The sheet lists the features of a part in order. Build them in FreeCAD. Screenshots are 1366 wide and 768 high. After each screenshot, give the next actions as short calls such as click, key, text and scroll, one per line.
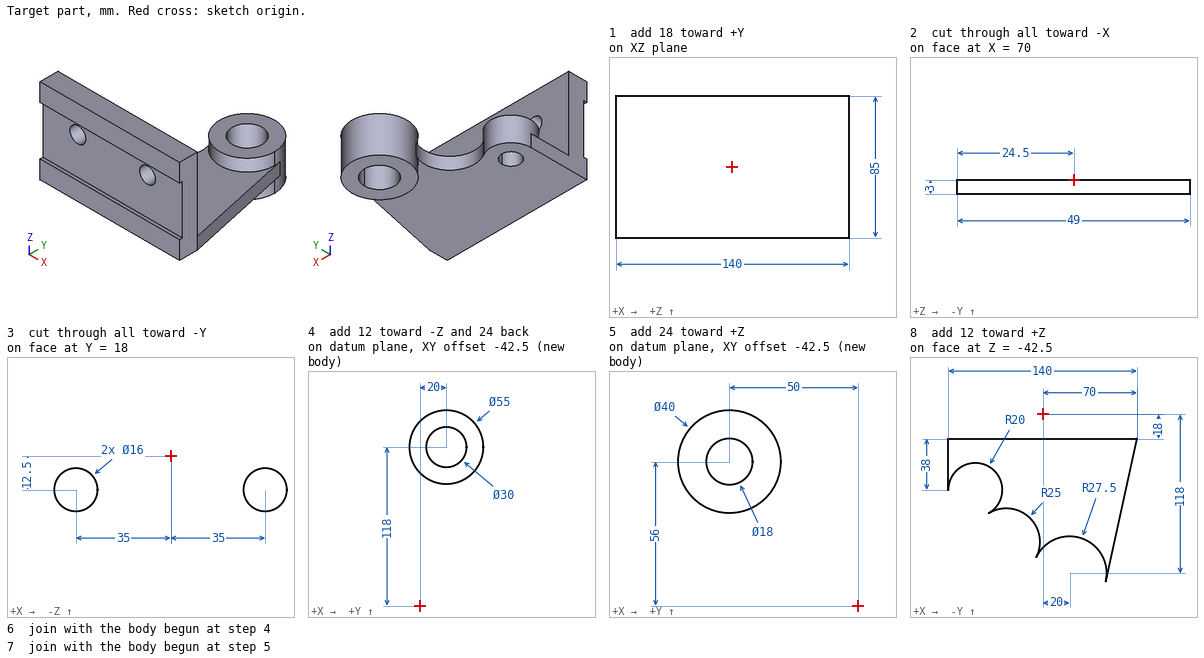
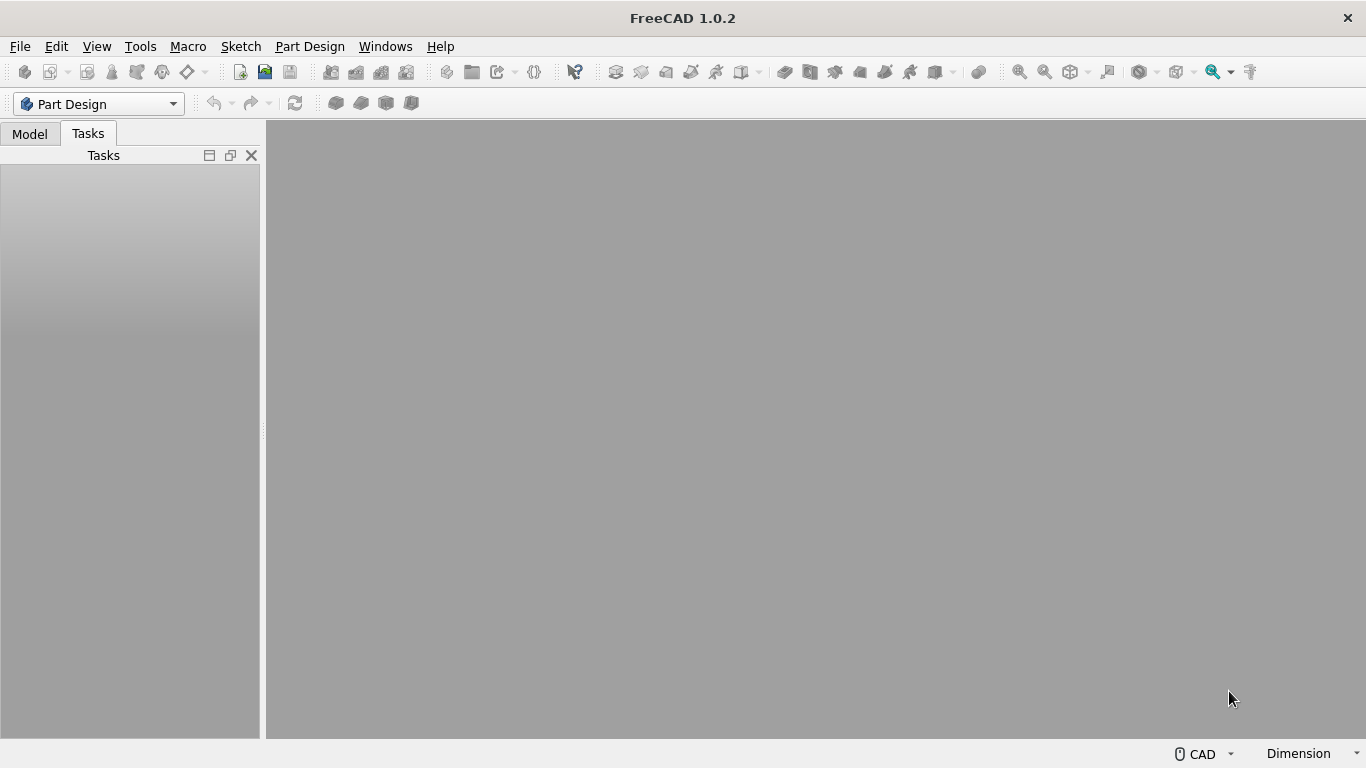
click(240, 72)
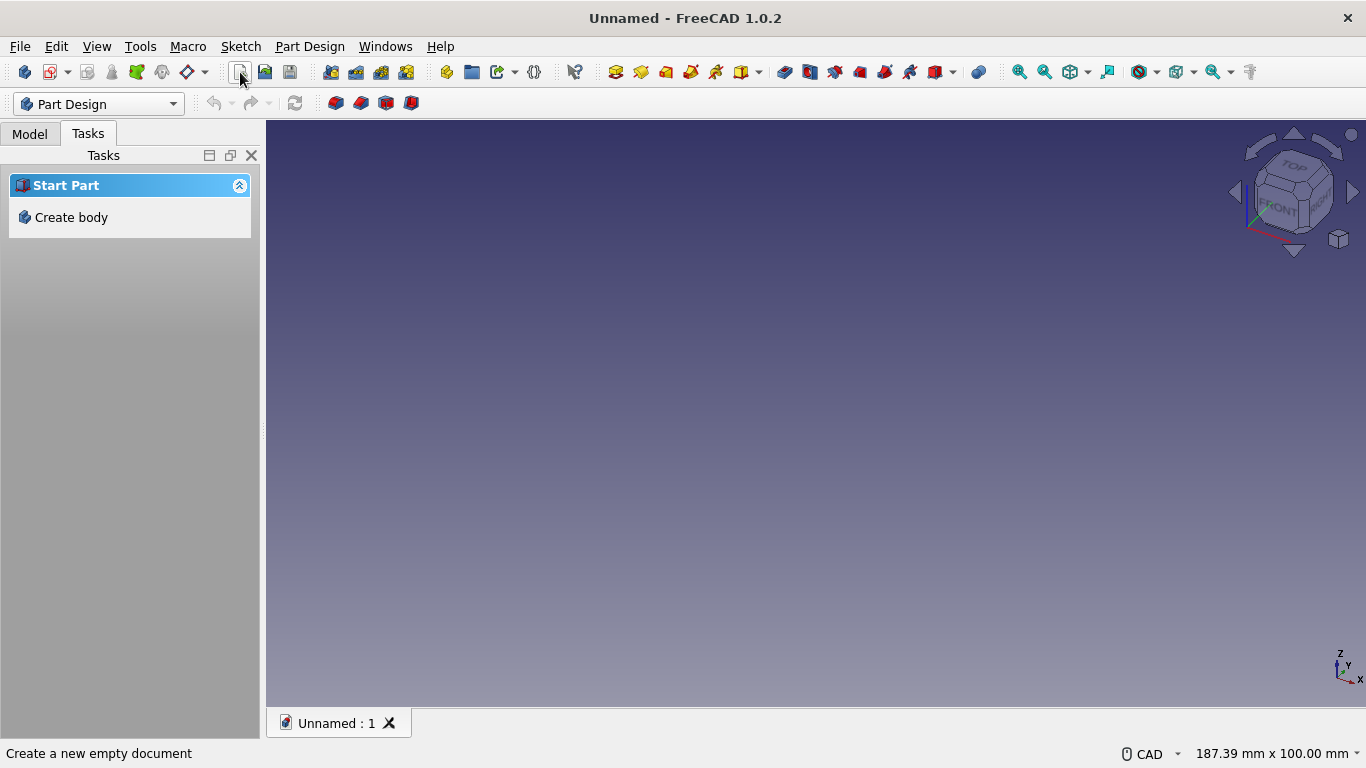
click(50, 72)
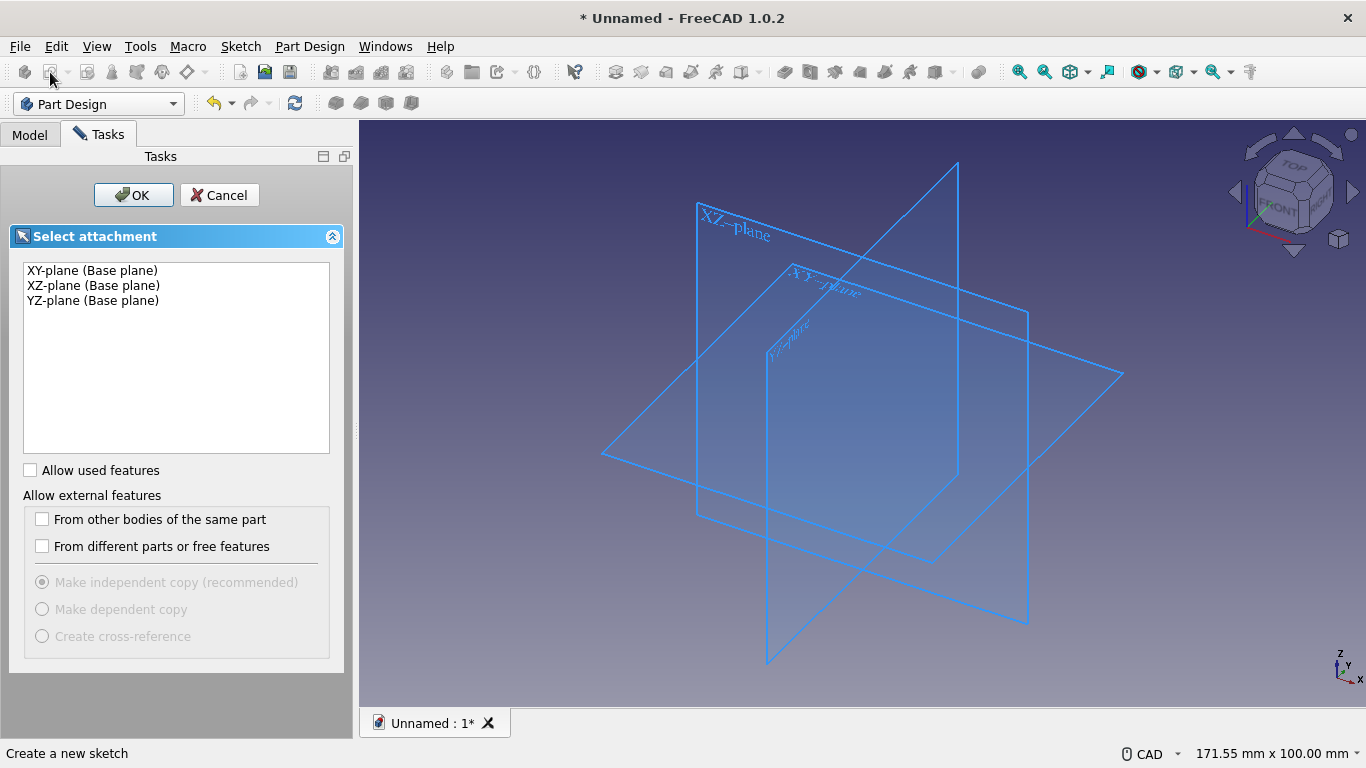
click(84, 286)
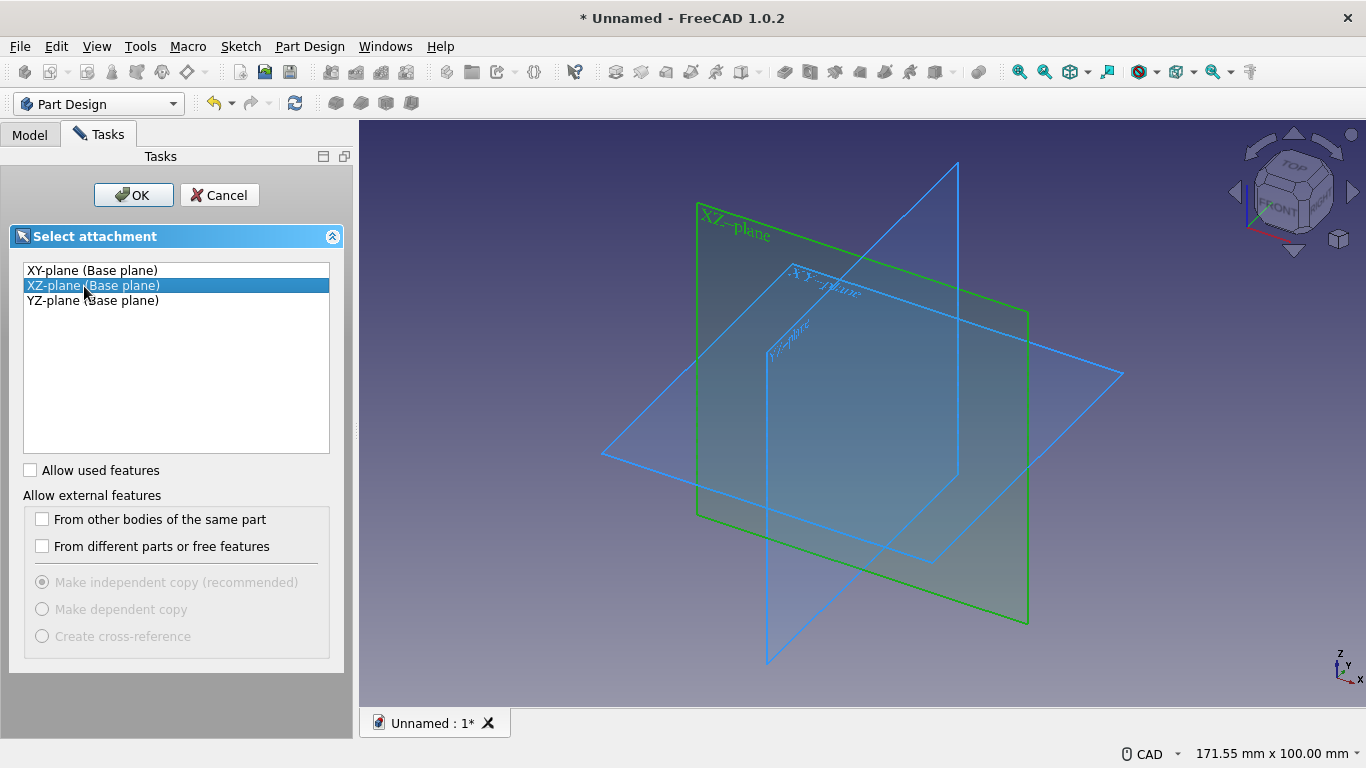
click(134, 195)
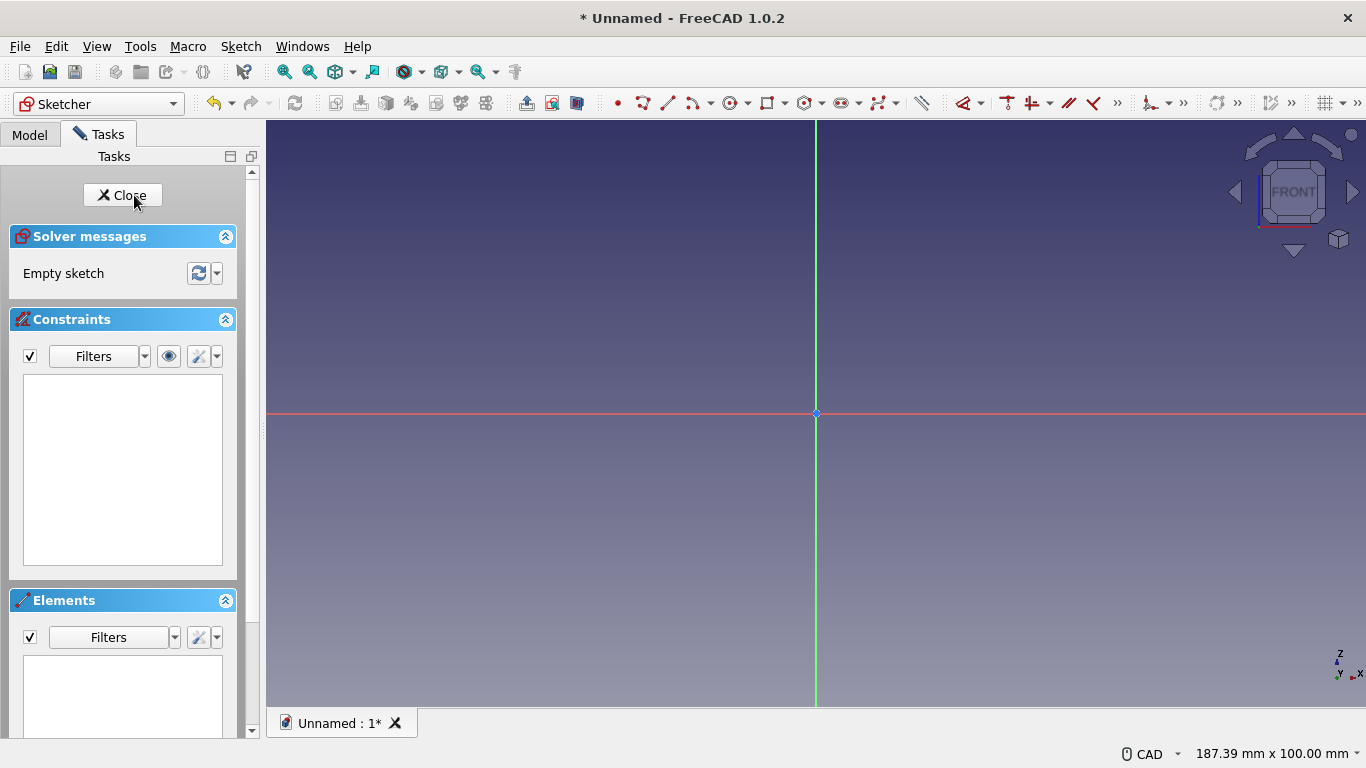
scroll(438, 413, down, 1)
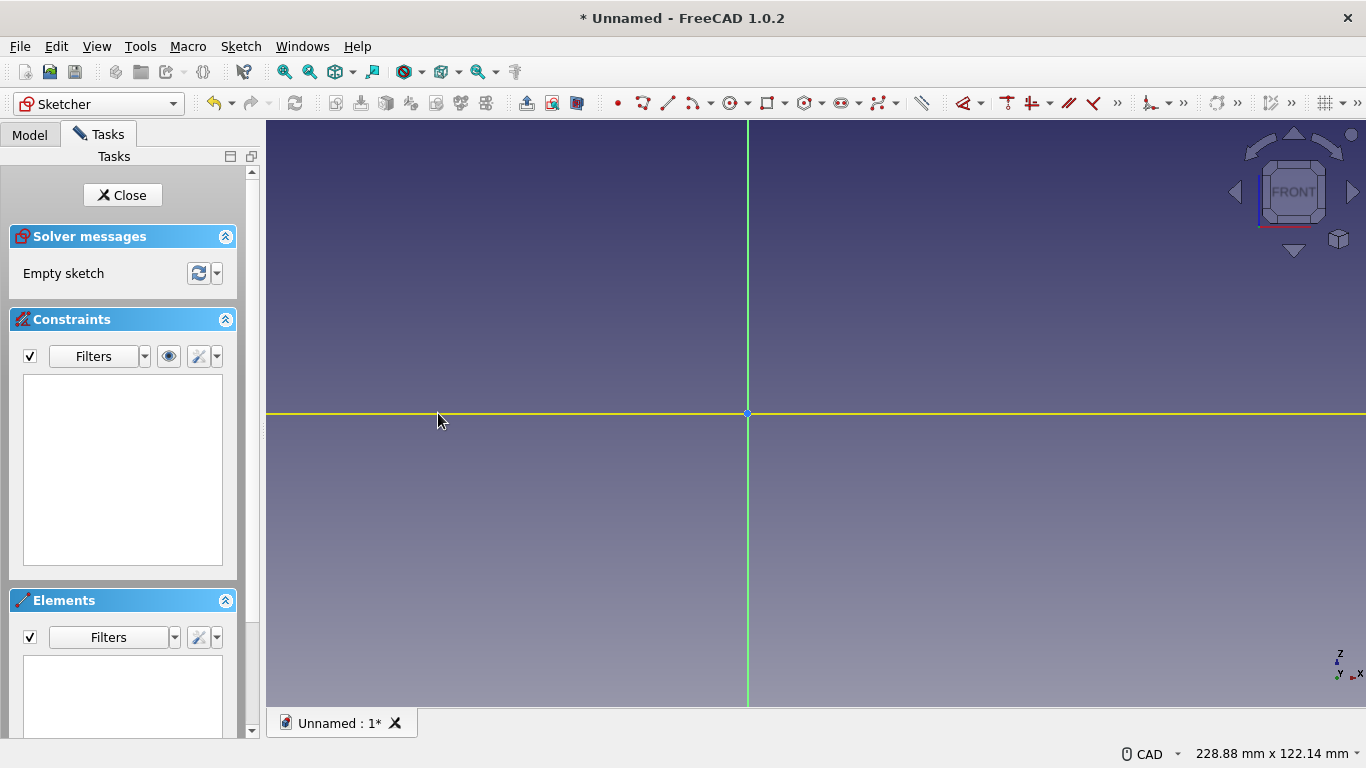
key(g)
key(v)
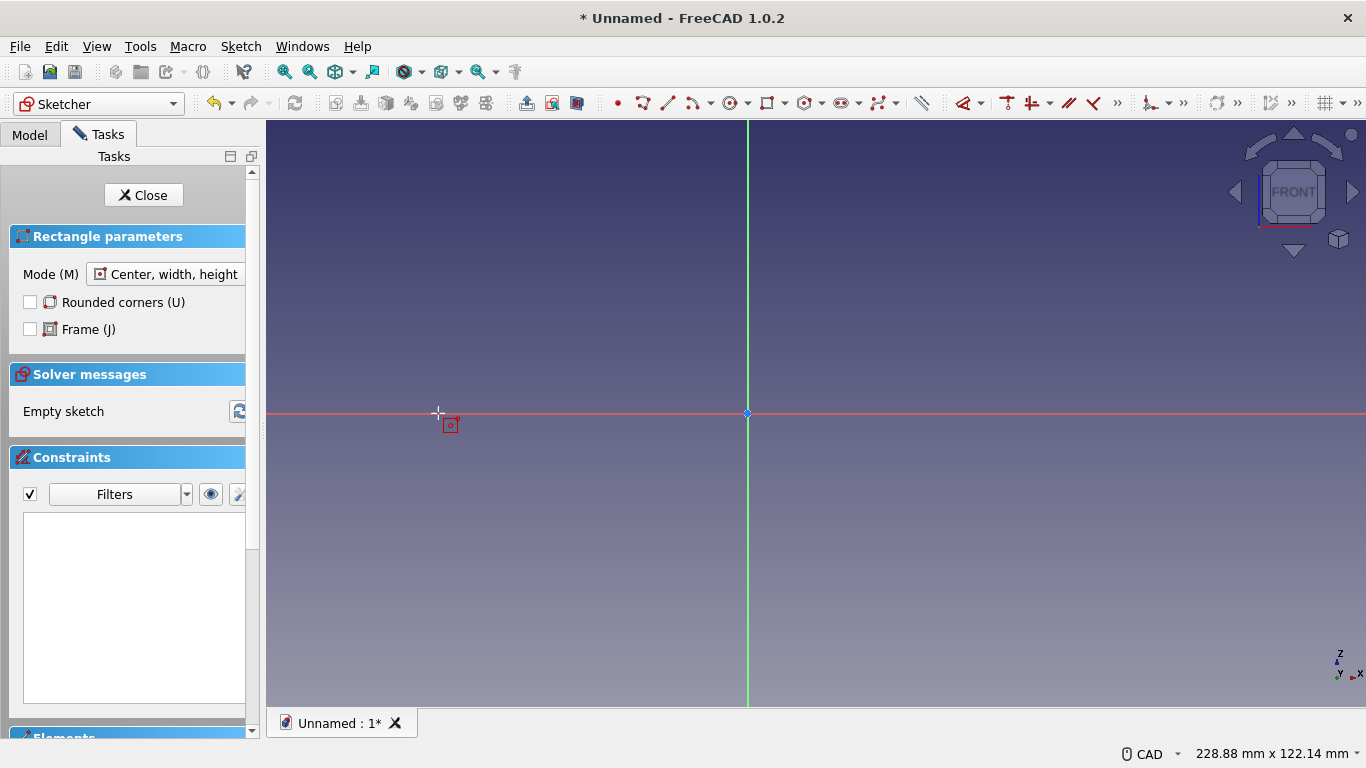
click(748, 414)
click(1084, 209)
key(Escape)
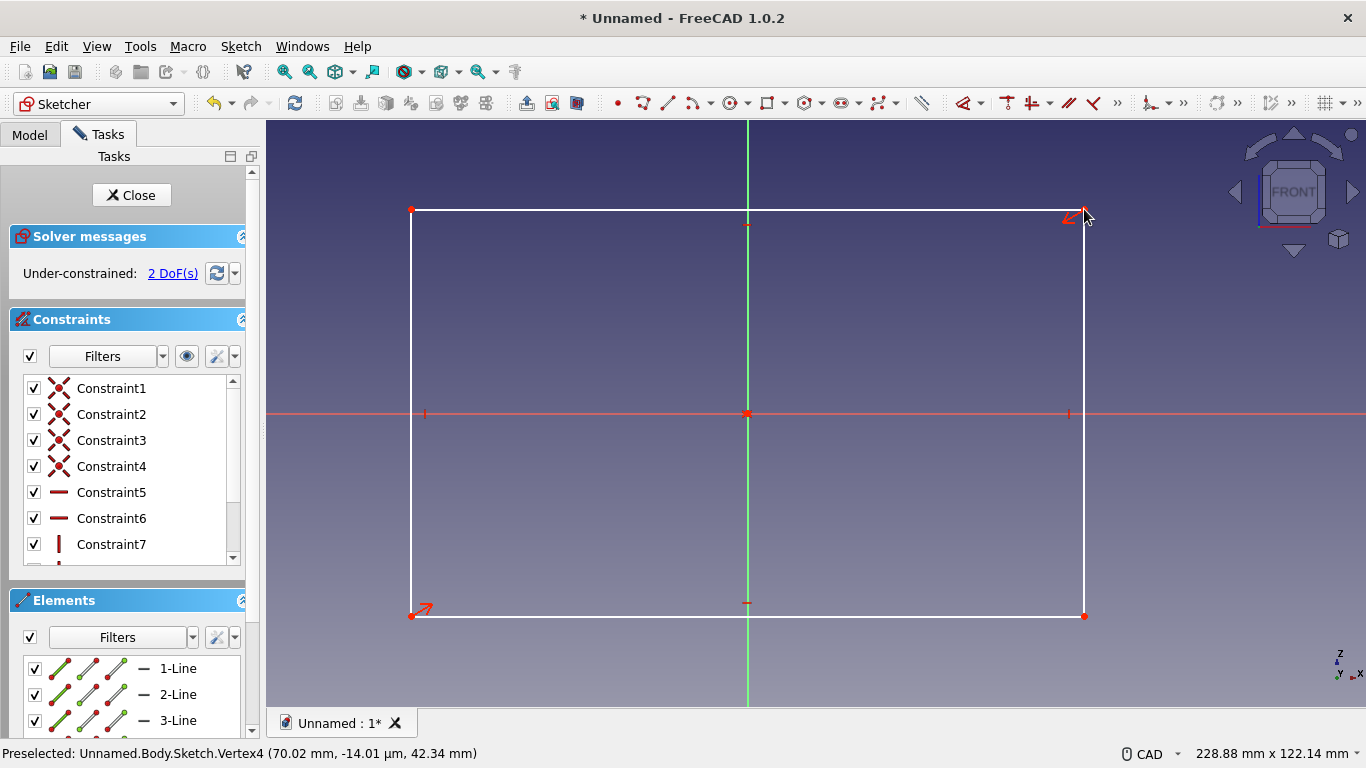
click(962, 104)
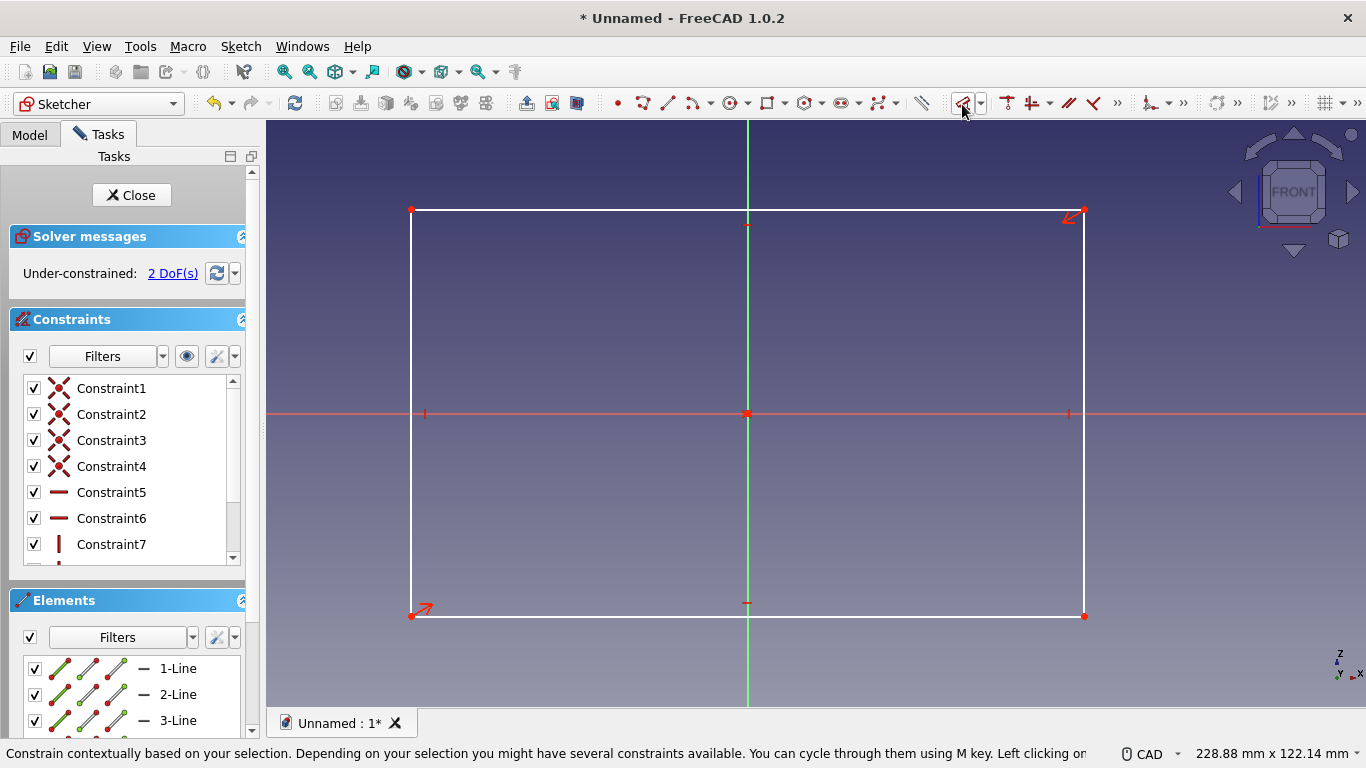
click(1084, 495)
click(1118, 320)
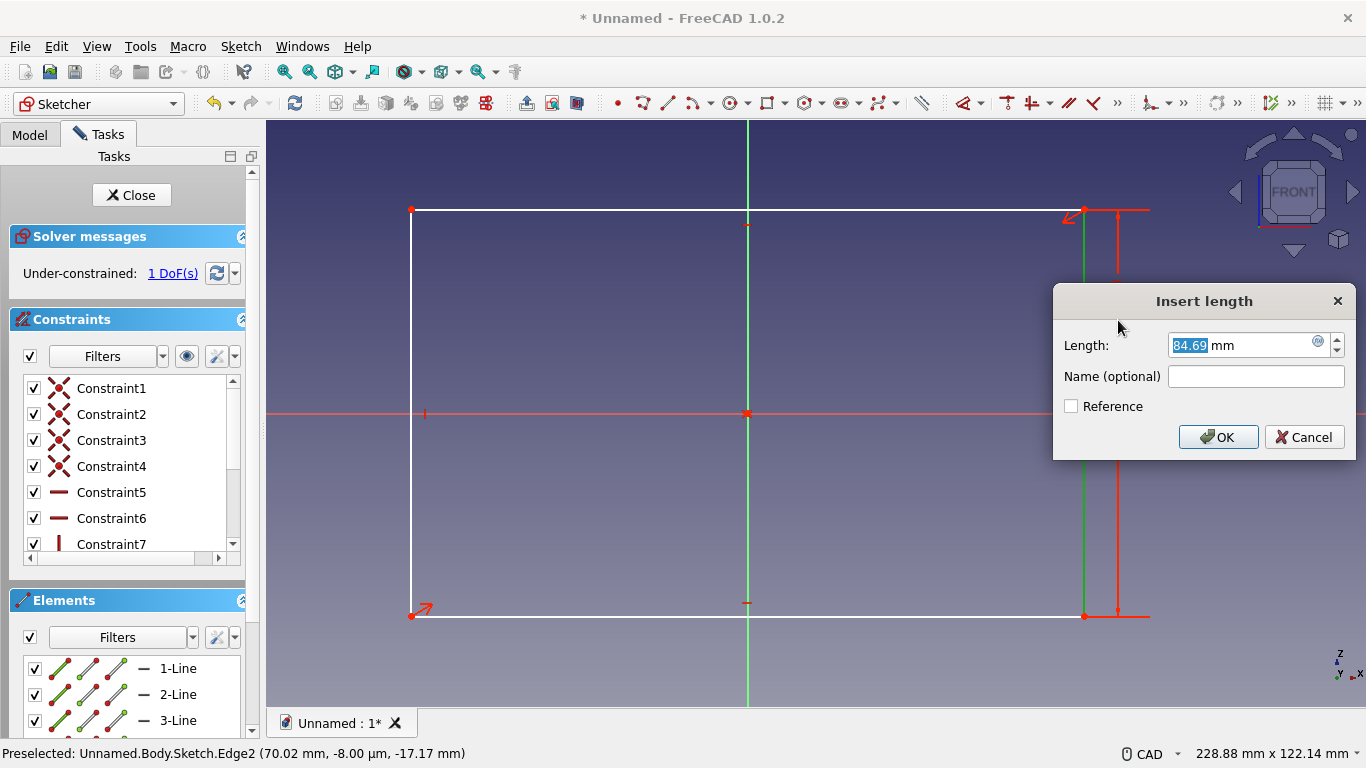
text(85)
key(Return)